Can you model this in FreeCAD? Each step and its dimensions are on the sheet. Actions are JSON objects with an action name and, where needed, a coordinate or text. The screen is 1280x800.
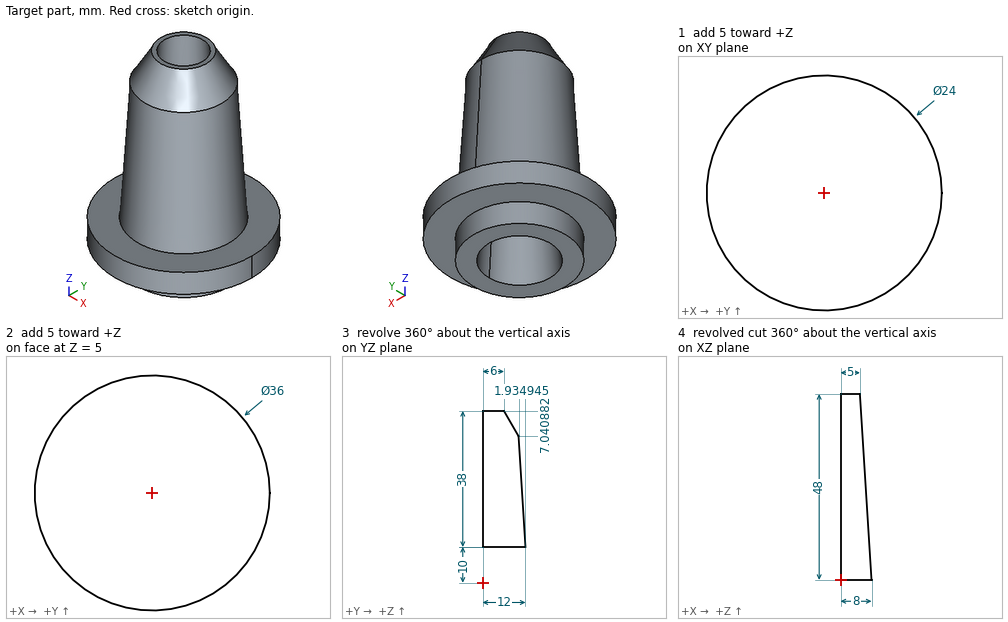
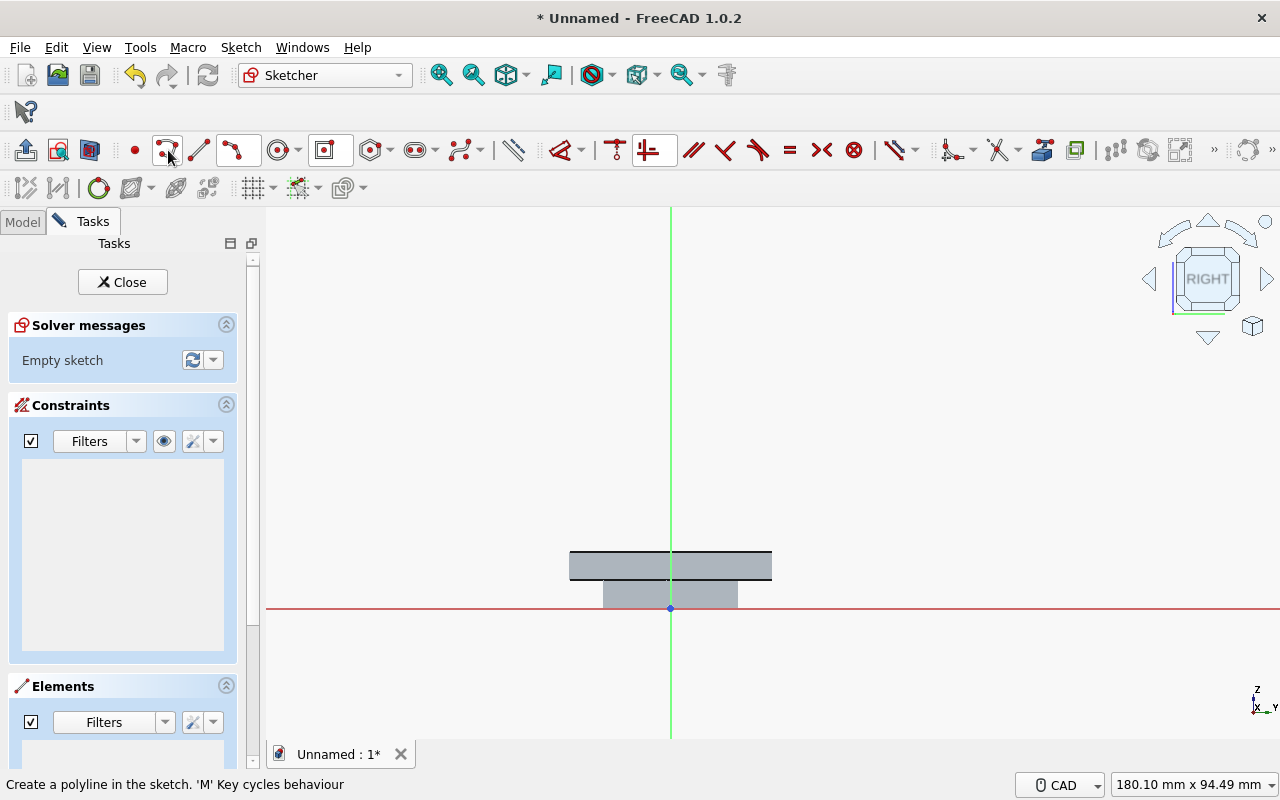
{"action": "left_click", "coordinate": [671, 552]}
{"action": "left_click", "coordinate": [738, 552]}
{"action": "left_click", "coordinate": [727, 378]}
{"action": "left_click", "coordinate": [704, 338]}
{"action": "left_click", "coordinate": [680, 338]}
{"action": "left_click", "coordinate": [671, 553]}
{"action": "key", "text": "Escape"}
{"action": "key", "text": "Escape"}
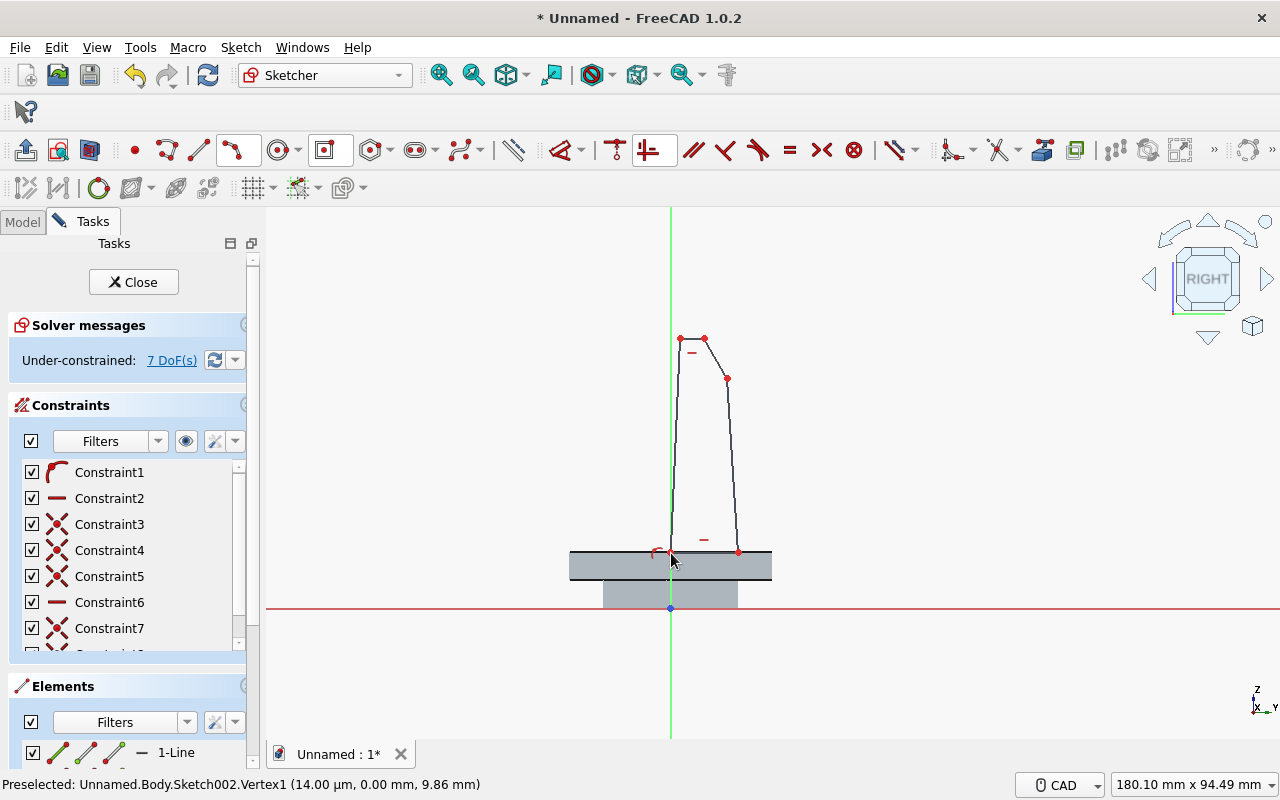
{"action": "left_click", "coordinate": [673, 489]}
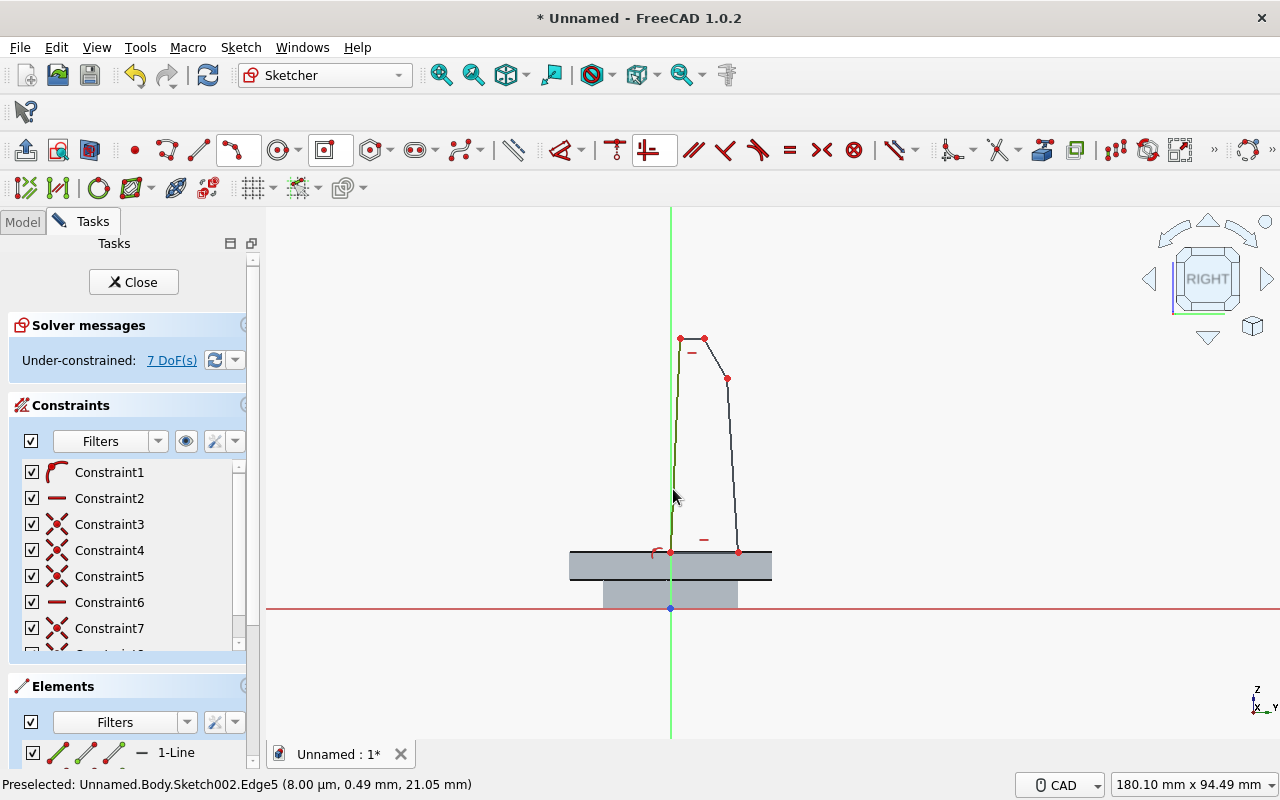
{"action": "left_click", "coordinate": [672, 150]}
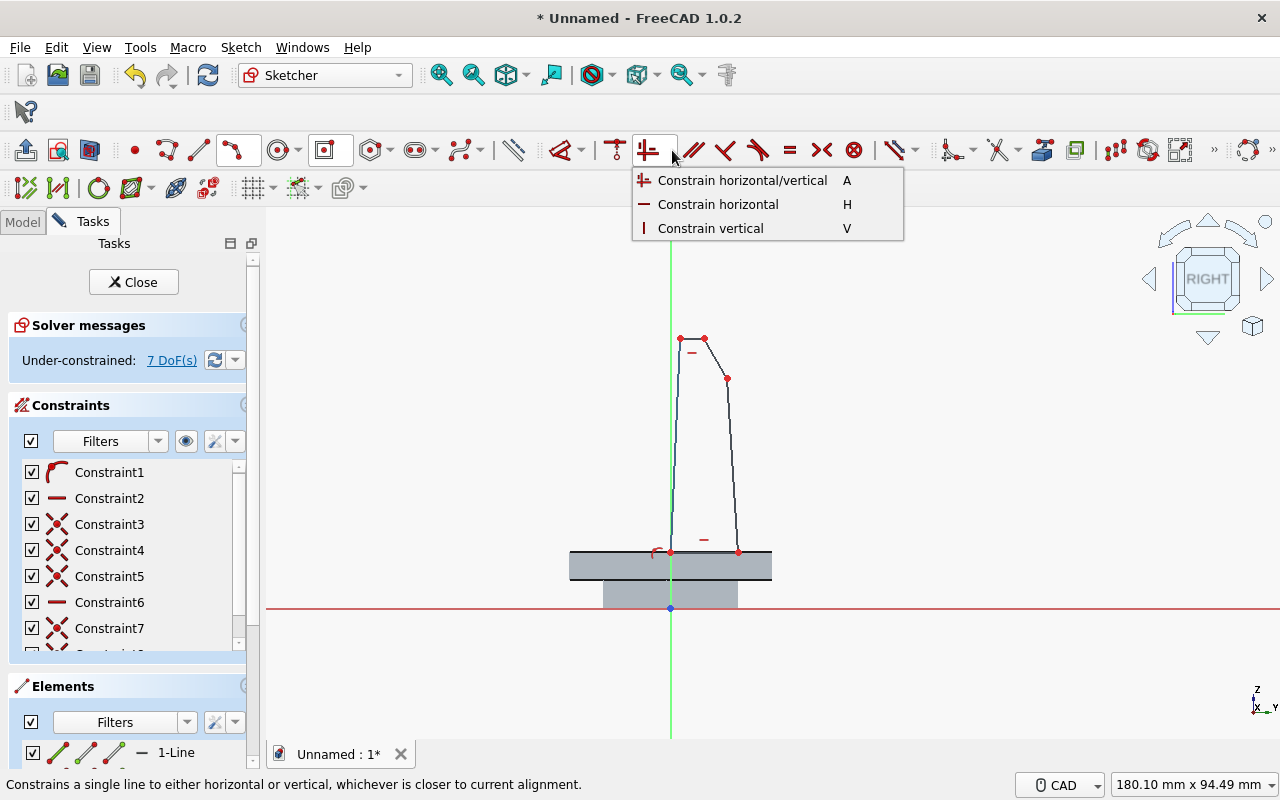
{"action": "left_click", "coordinate": [768, 228]}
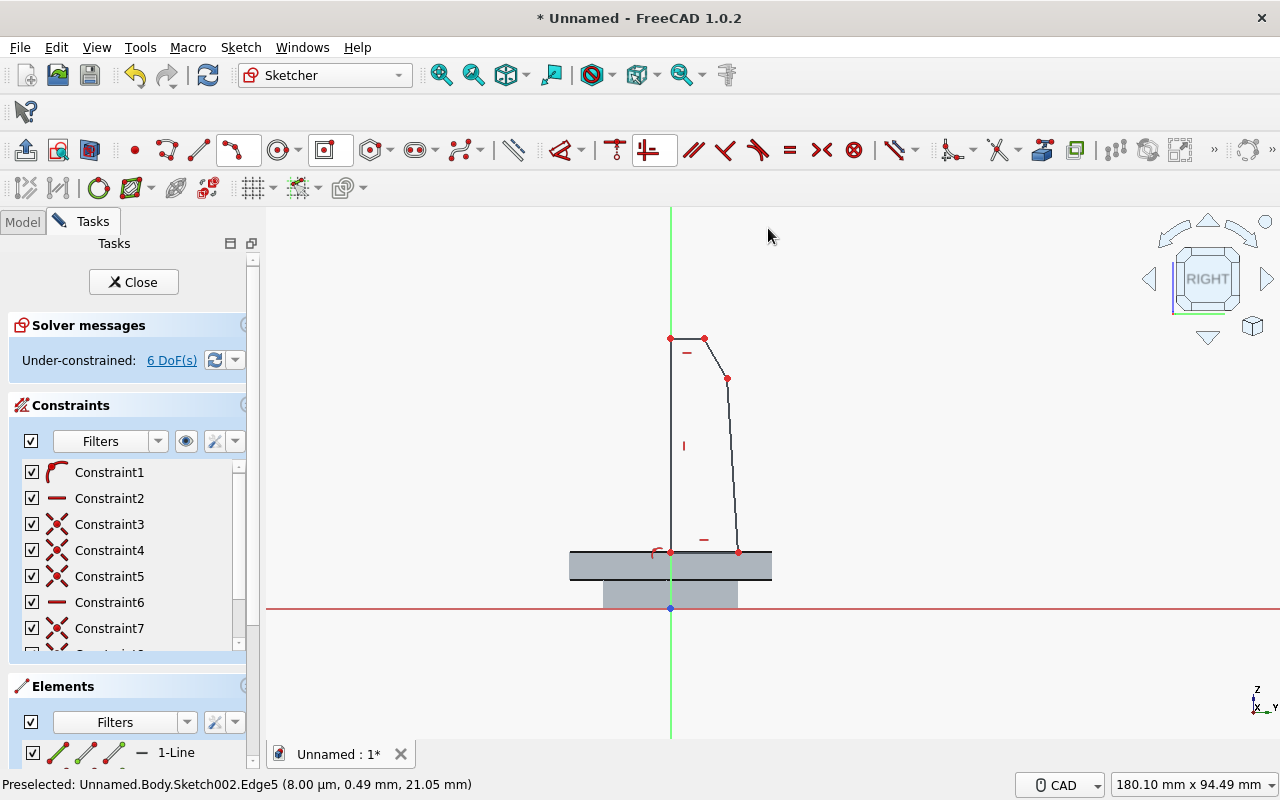
{"action": "left_click", "coordinate": [560, 150]}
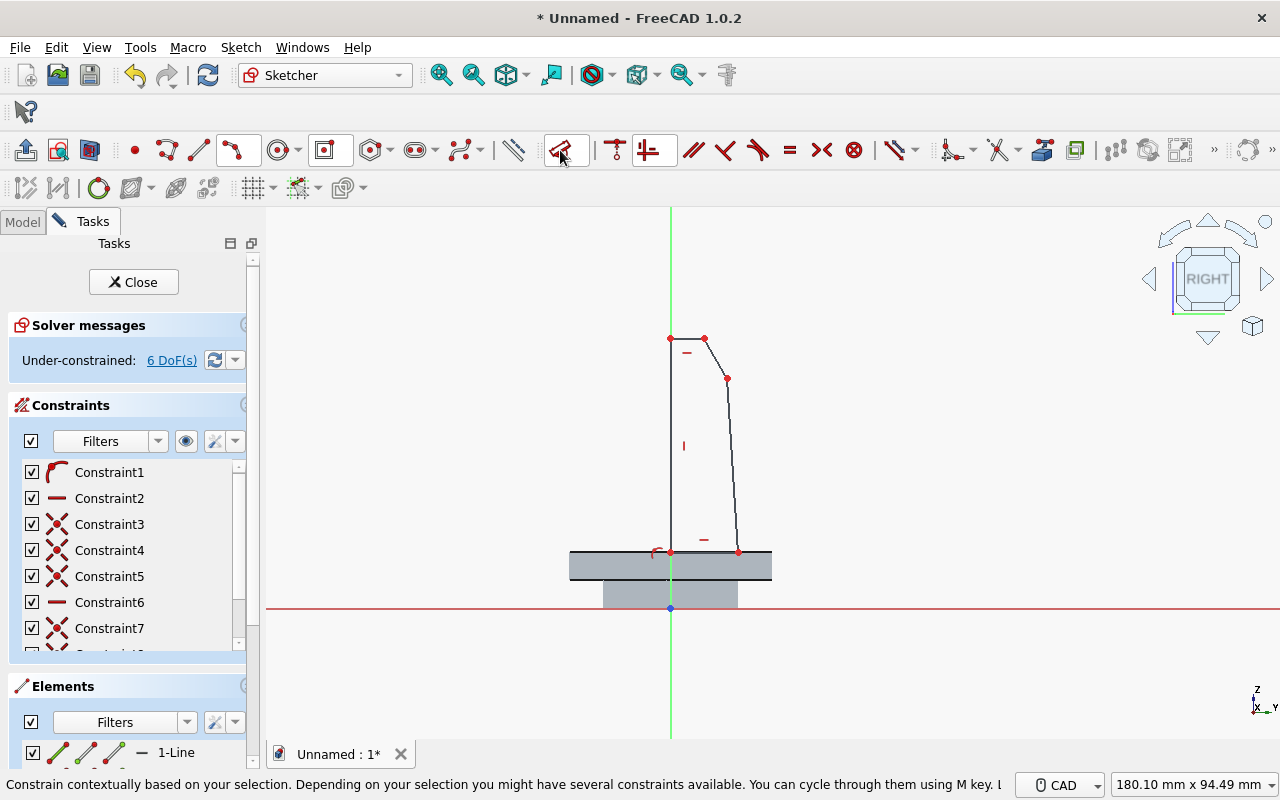
{"action": "scroll", "coordinate": [694, 339], "scroll_direction": "up", "scroll_amount": 2}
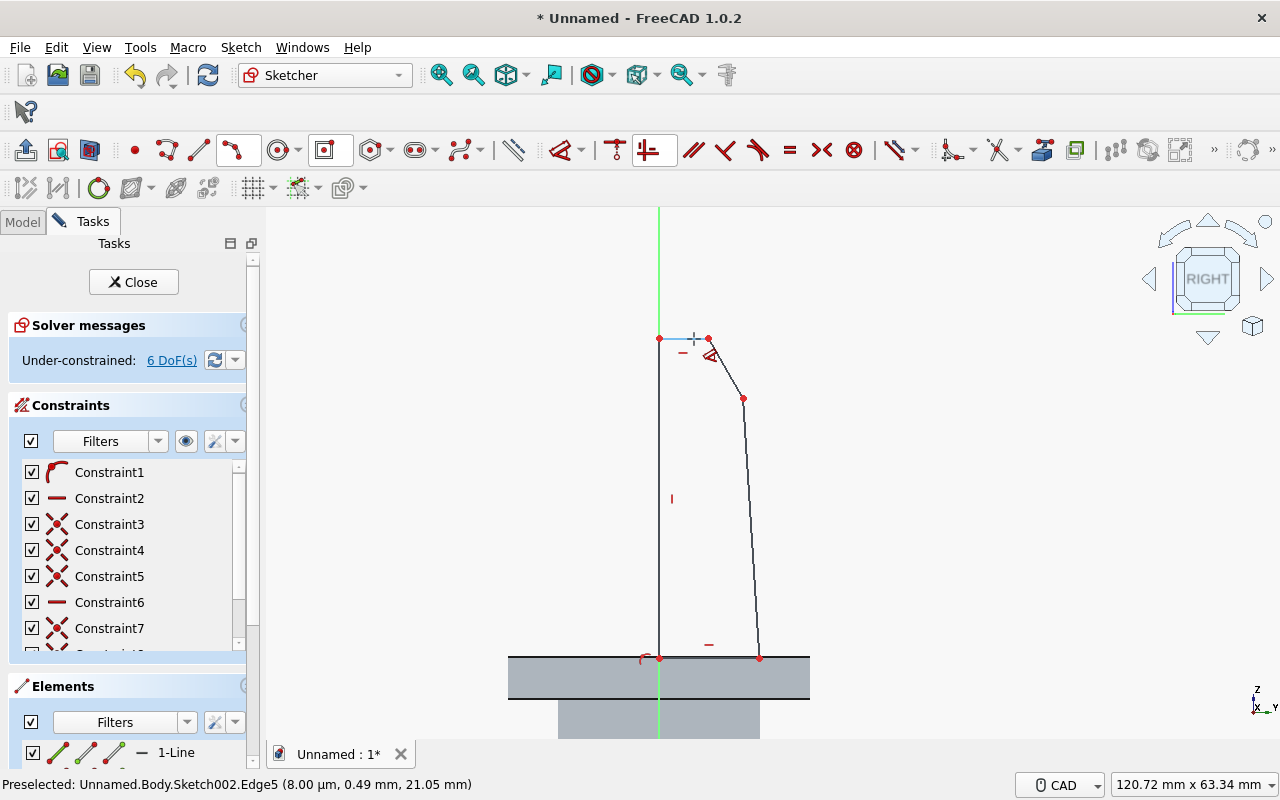
{"action": "left_click", "coordinate": [694, 339]}
{"action": "left_click", "coordinate": [684, 305]}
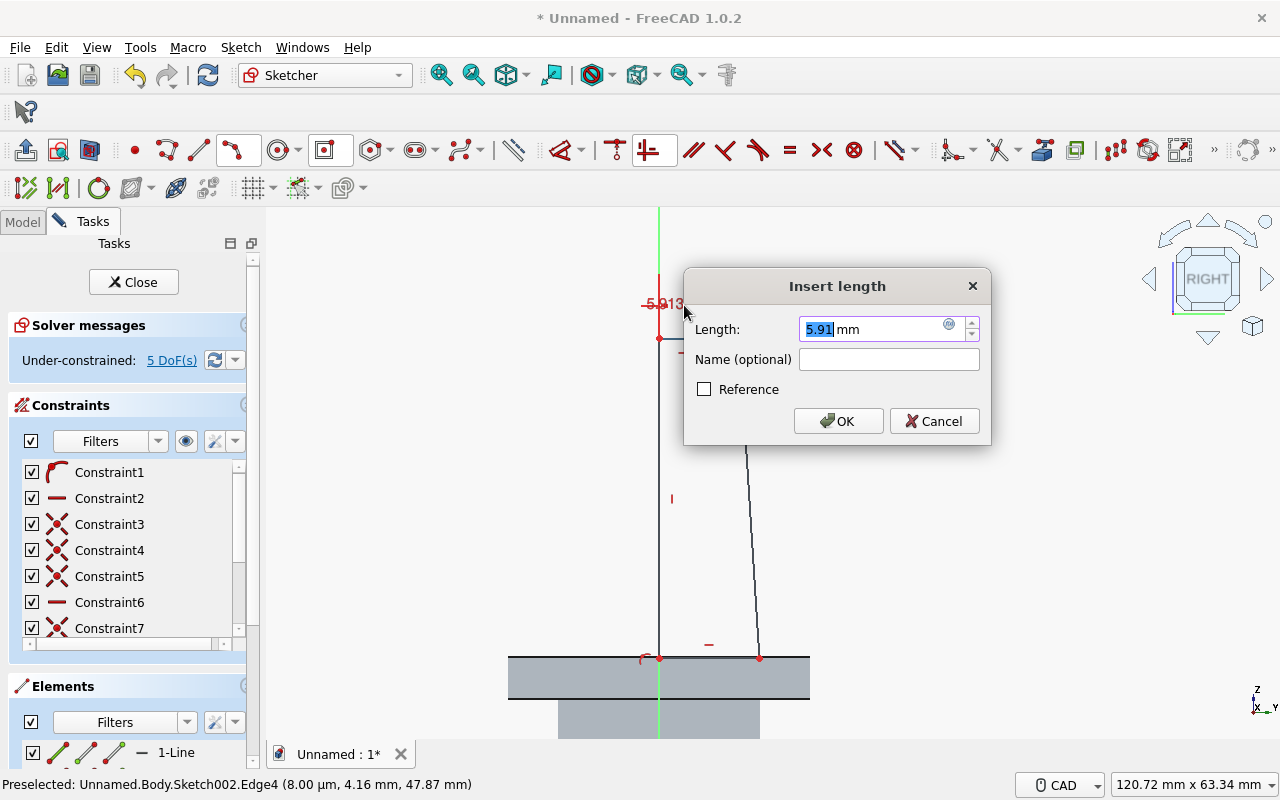
{"action": "type", "text": "6"}
{"action": "key", "text": "Return"}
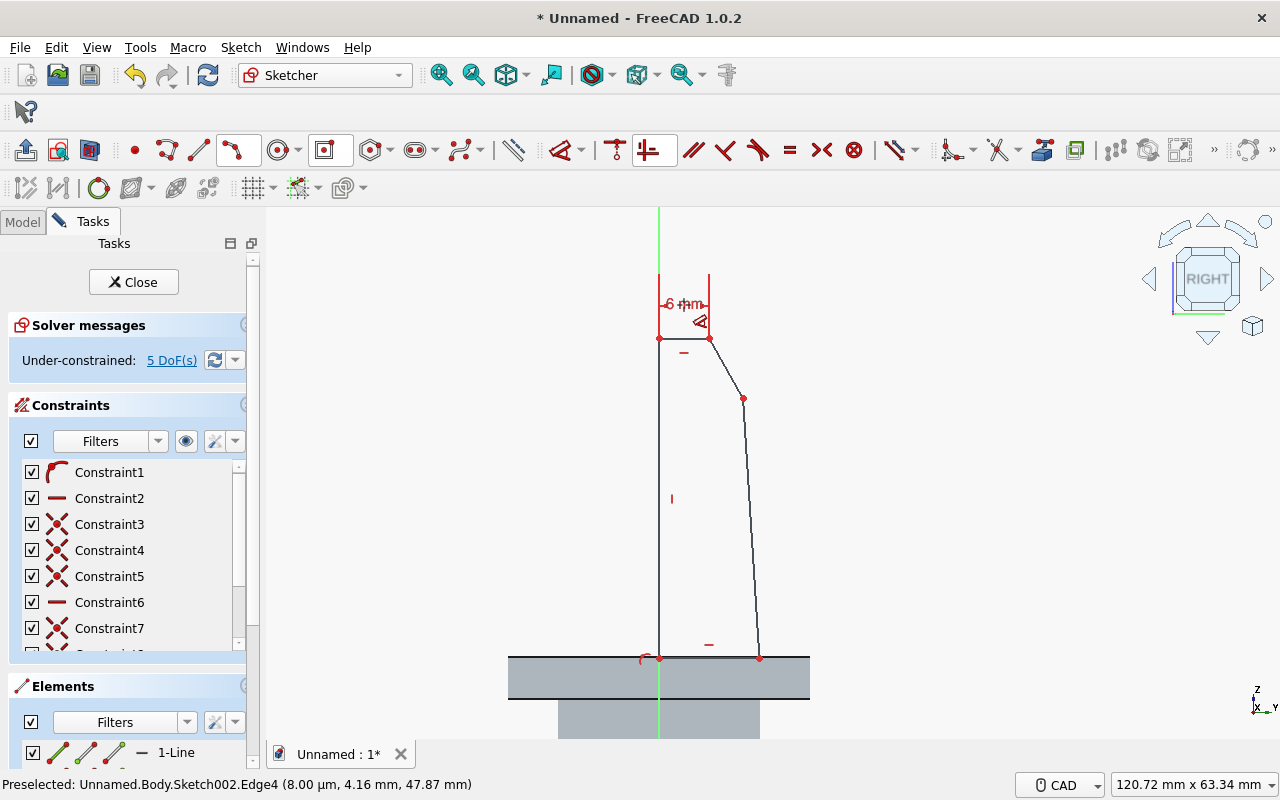
{"action": "left_click", "coordinate": [689, 658]}
{"action": "left_click", "coordinate": [709, 692]}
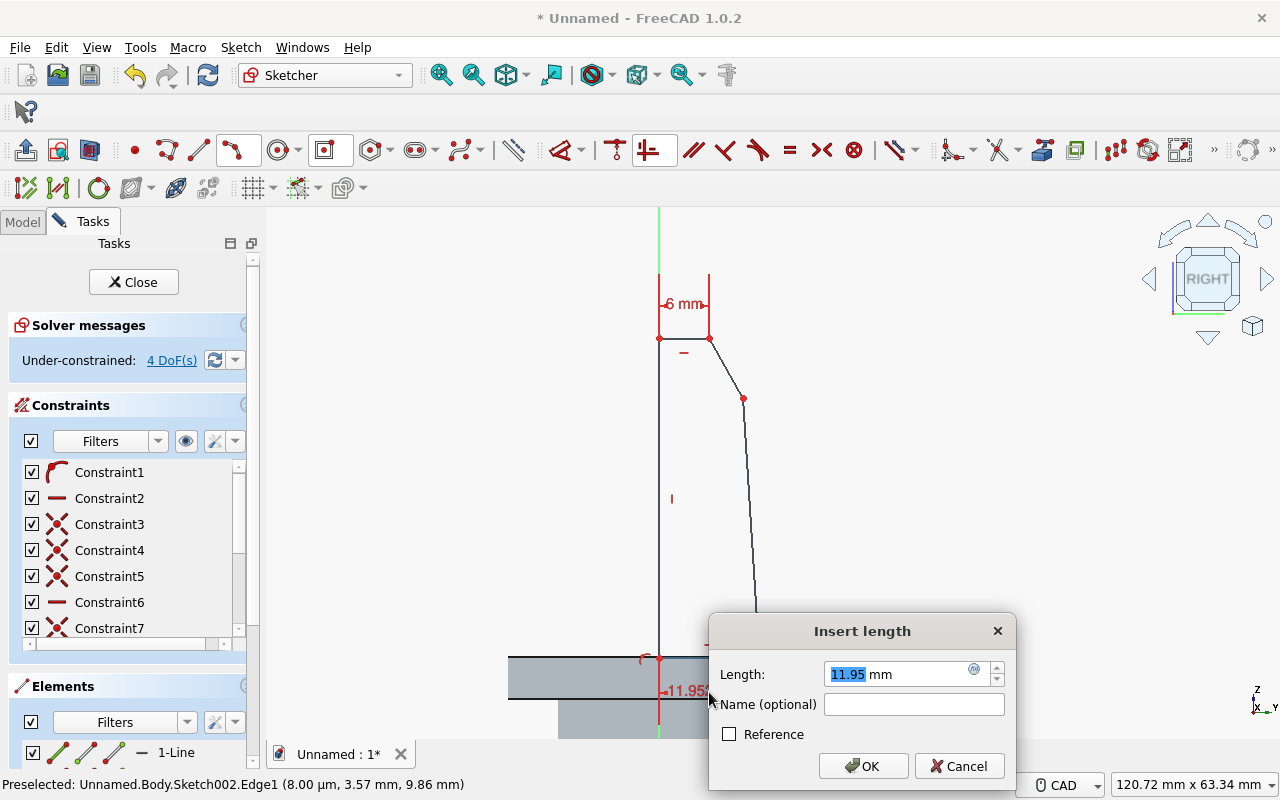
{"action": "type", "text": "12"}
{"action": "key", "text": "Return"}